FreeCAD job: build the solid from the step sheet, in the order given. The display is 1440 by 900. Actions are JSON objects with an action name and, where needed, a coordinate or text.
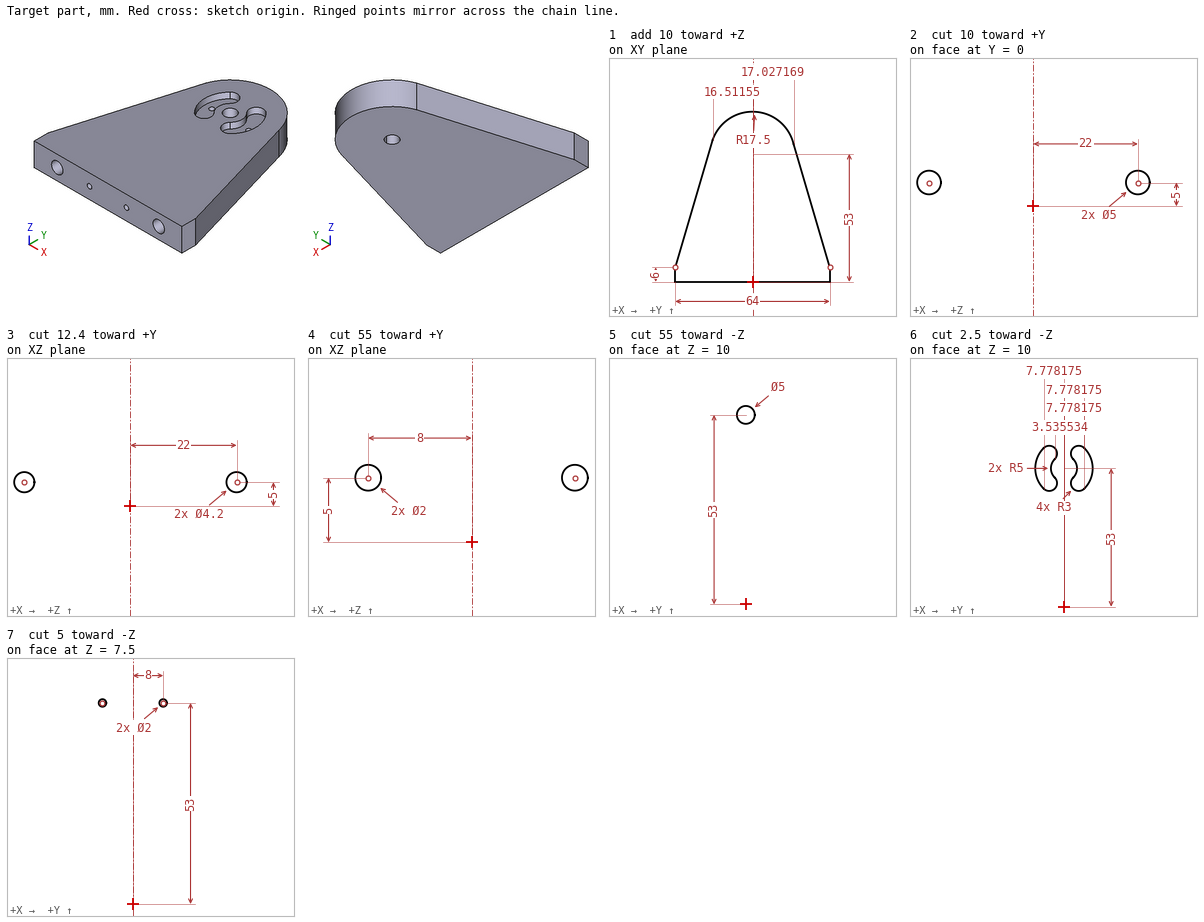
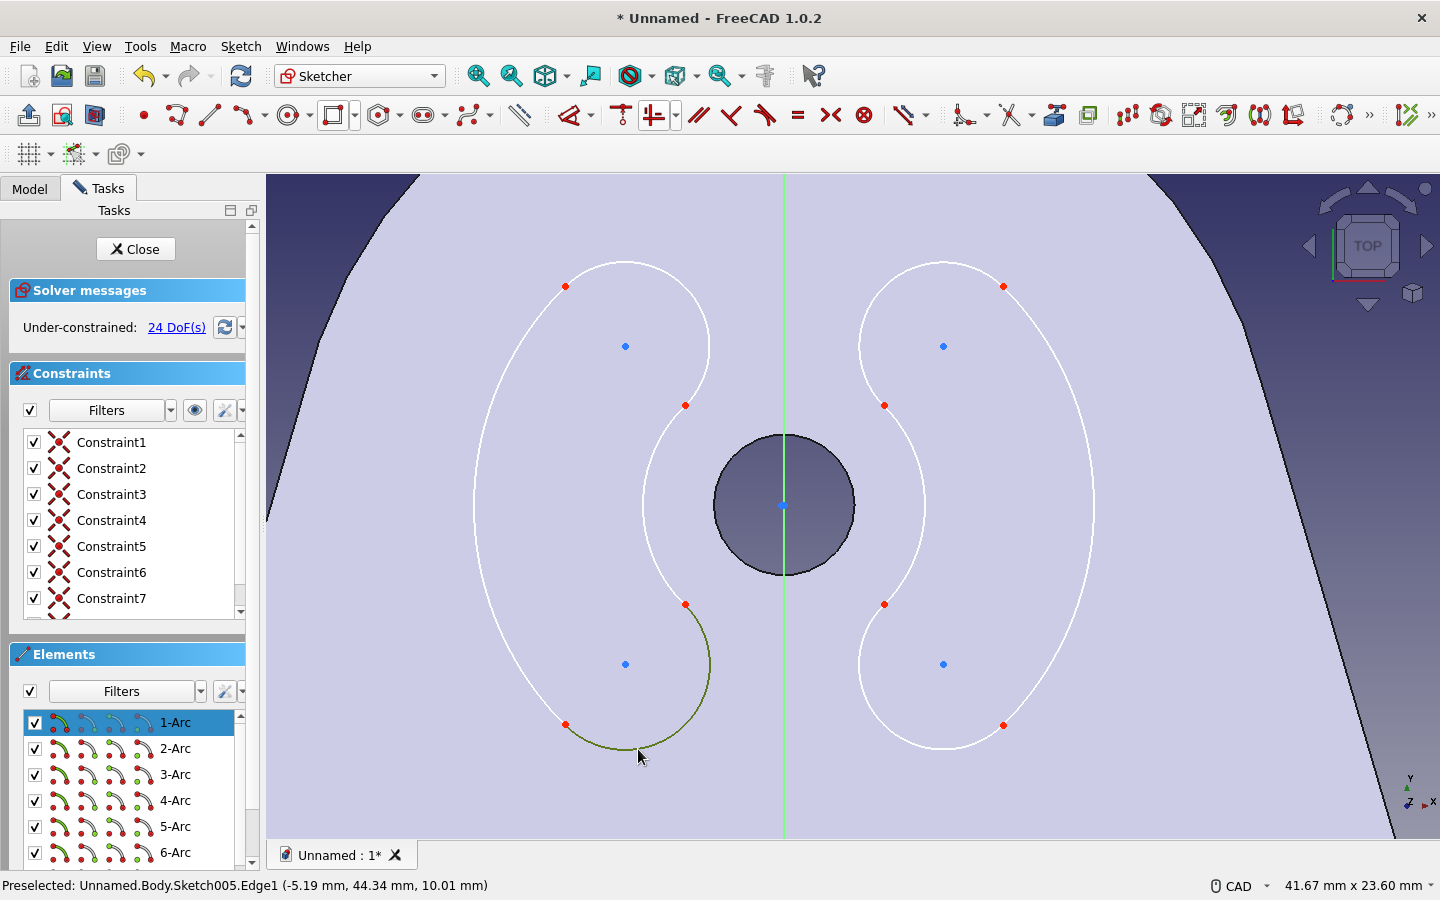
{"action": "left_click", "coordinate": [650, 462]}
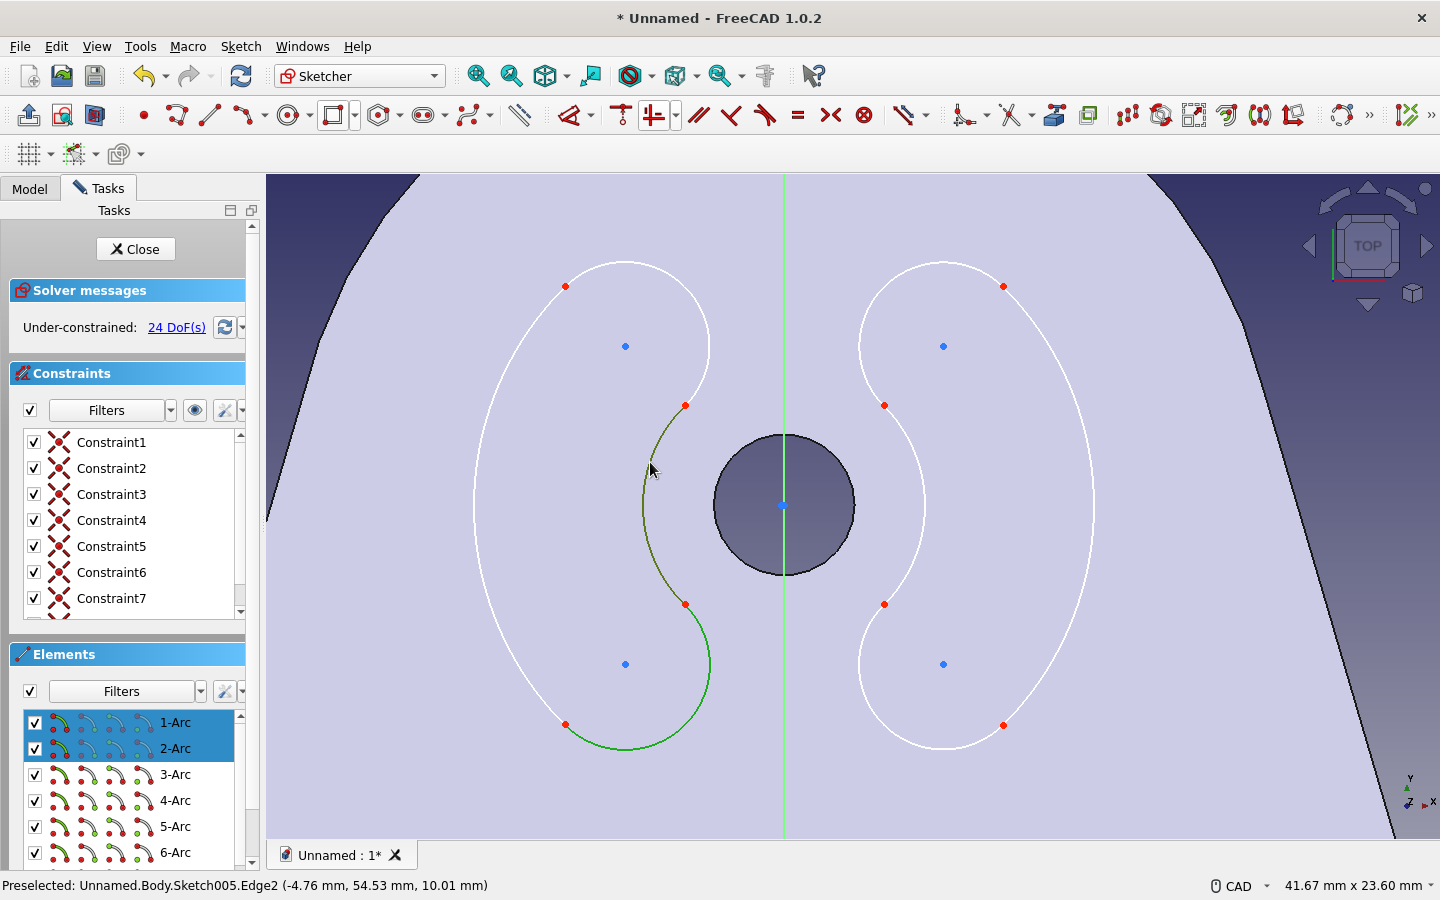
{"action": "left_click", "coordinate": [765, 116]}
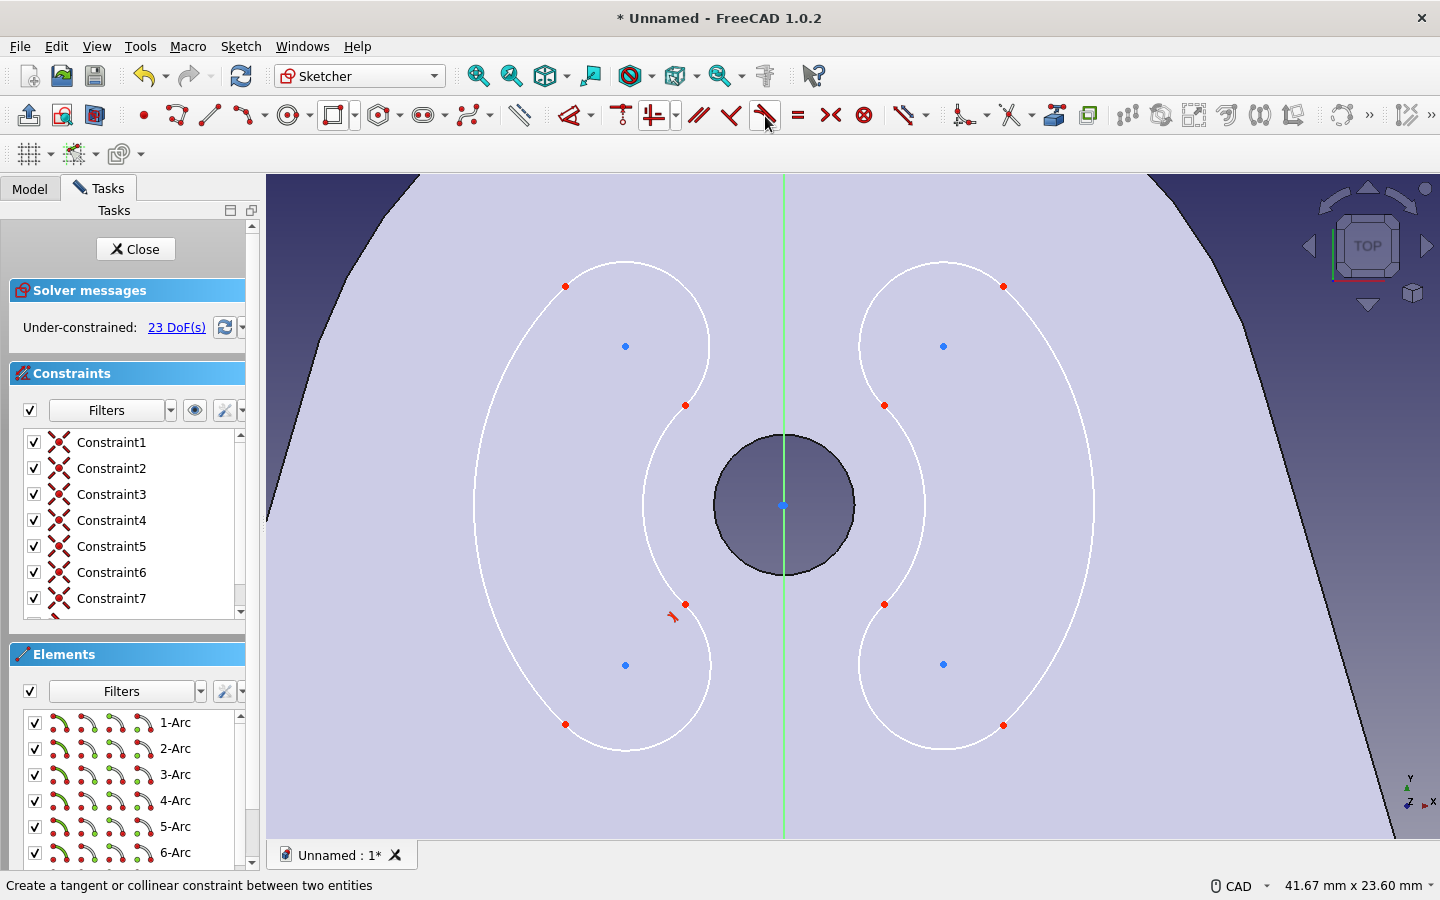
{"action": "left_click", "coordinate": [639, 750]}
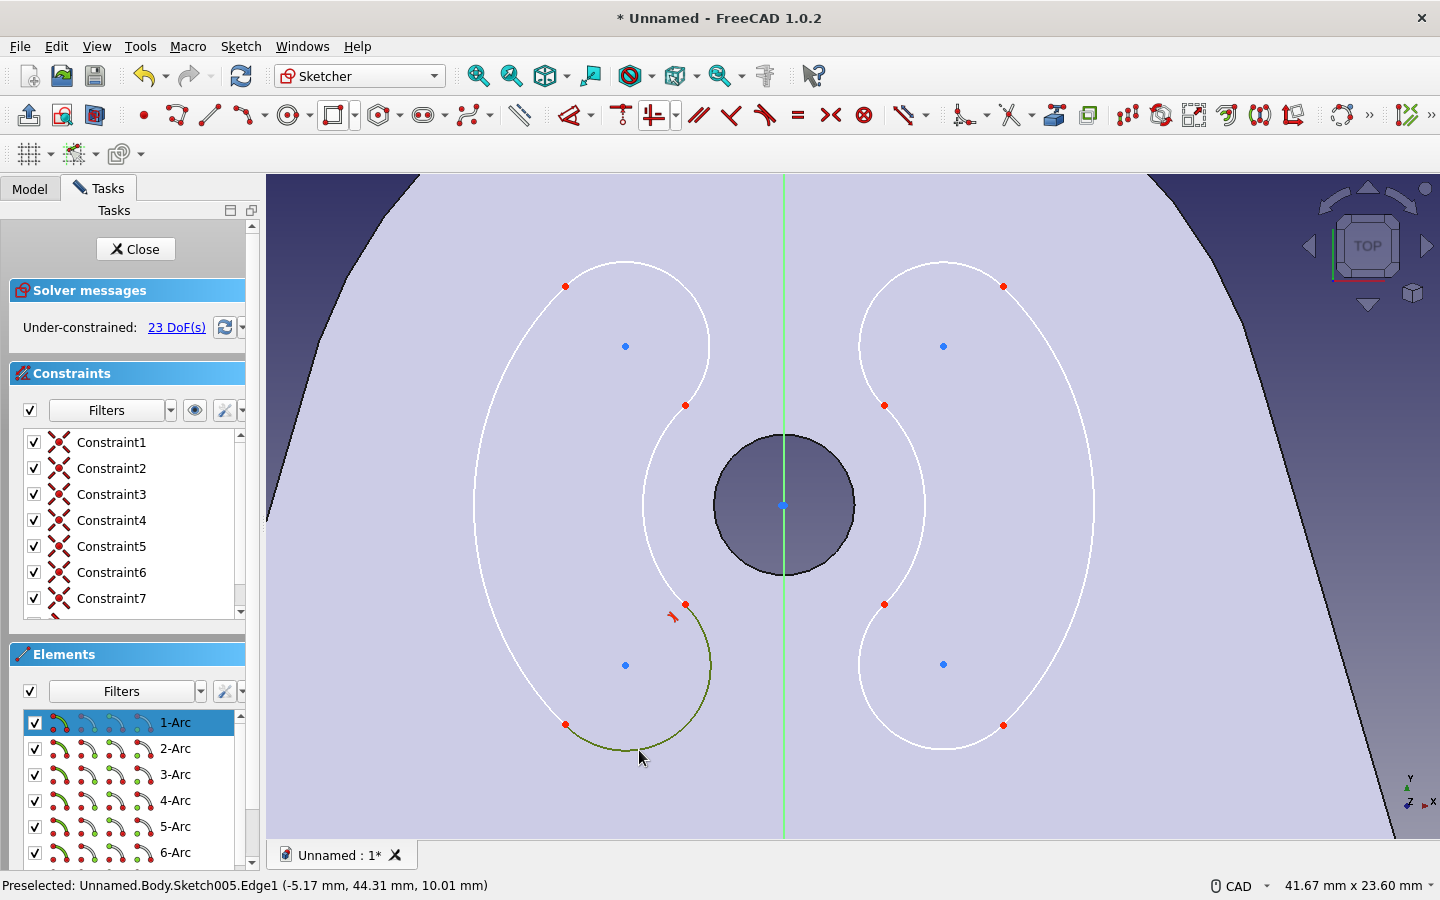
{"action": "left_click", "coordinate": [489, 410]}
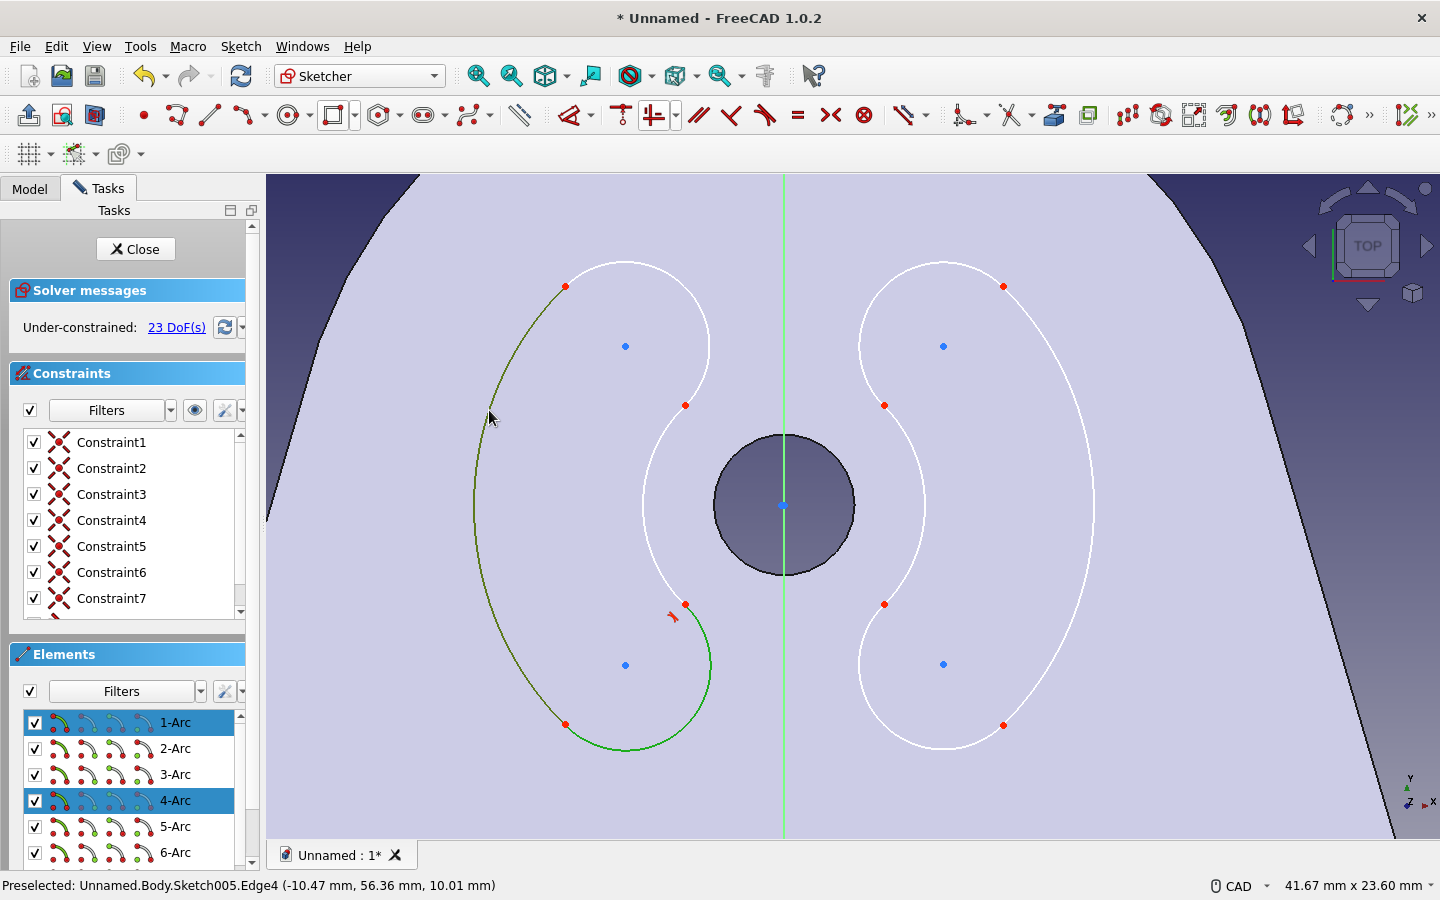
{"action": "left_click", "coordinate": [765, 116]}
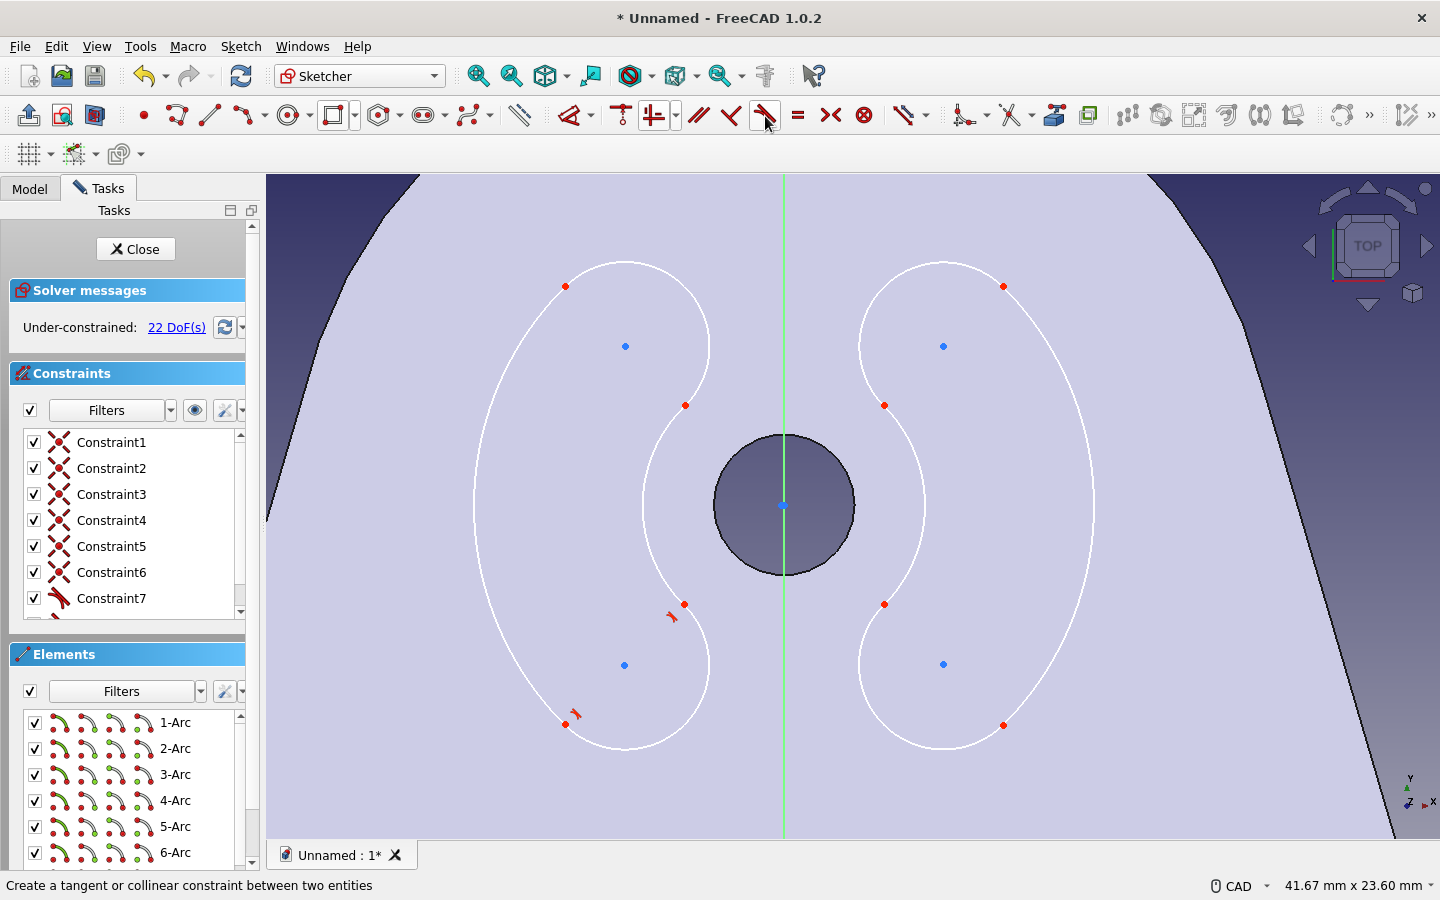
{"action": "left_click", "coordinate": [650, 462]}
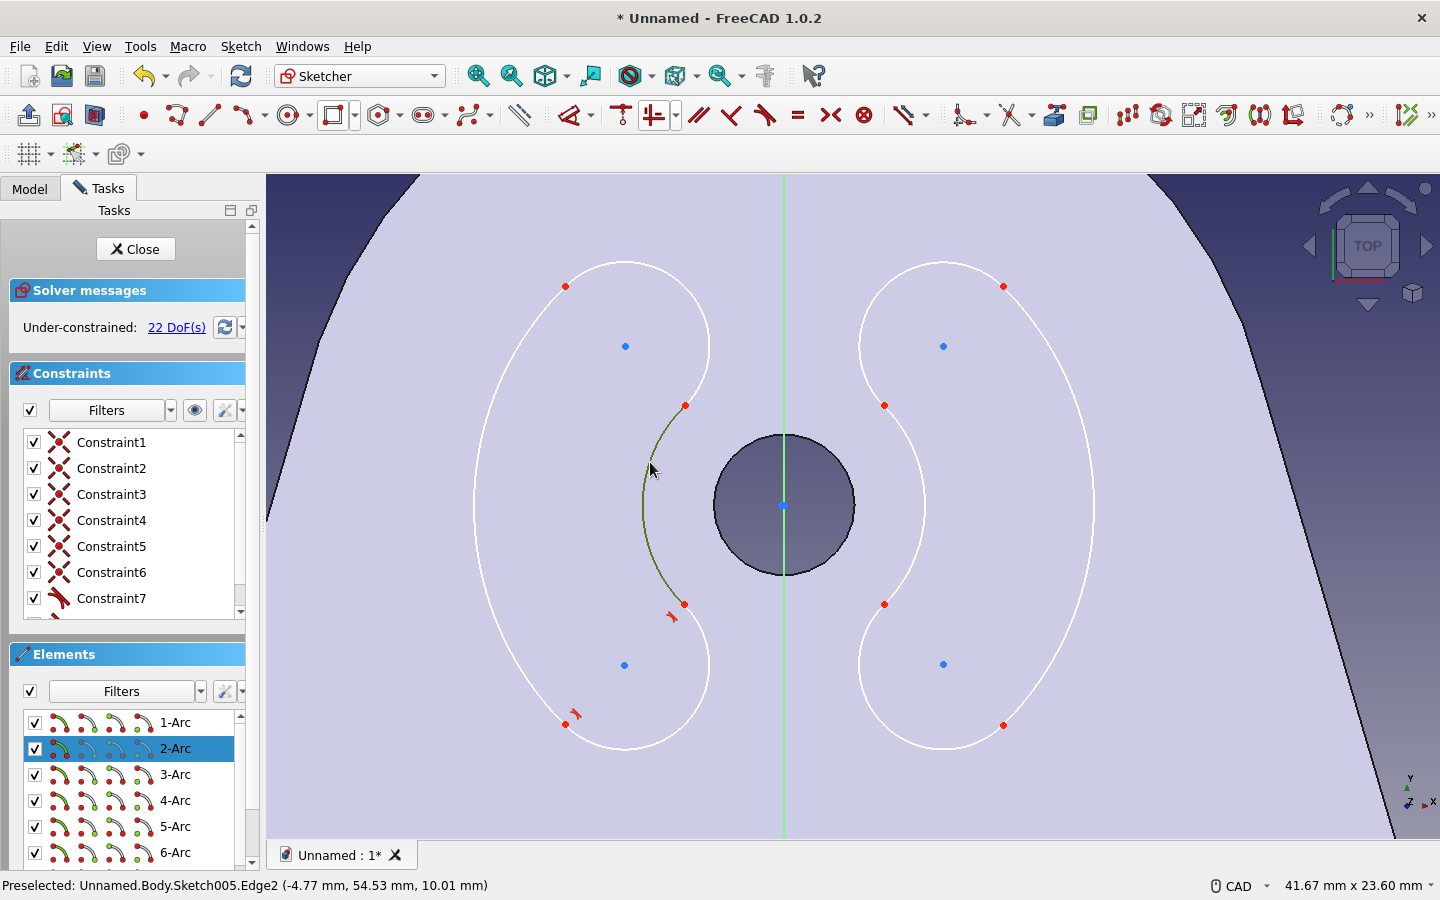
{"action": "left_click", "coordinate": [708, 333]}